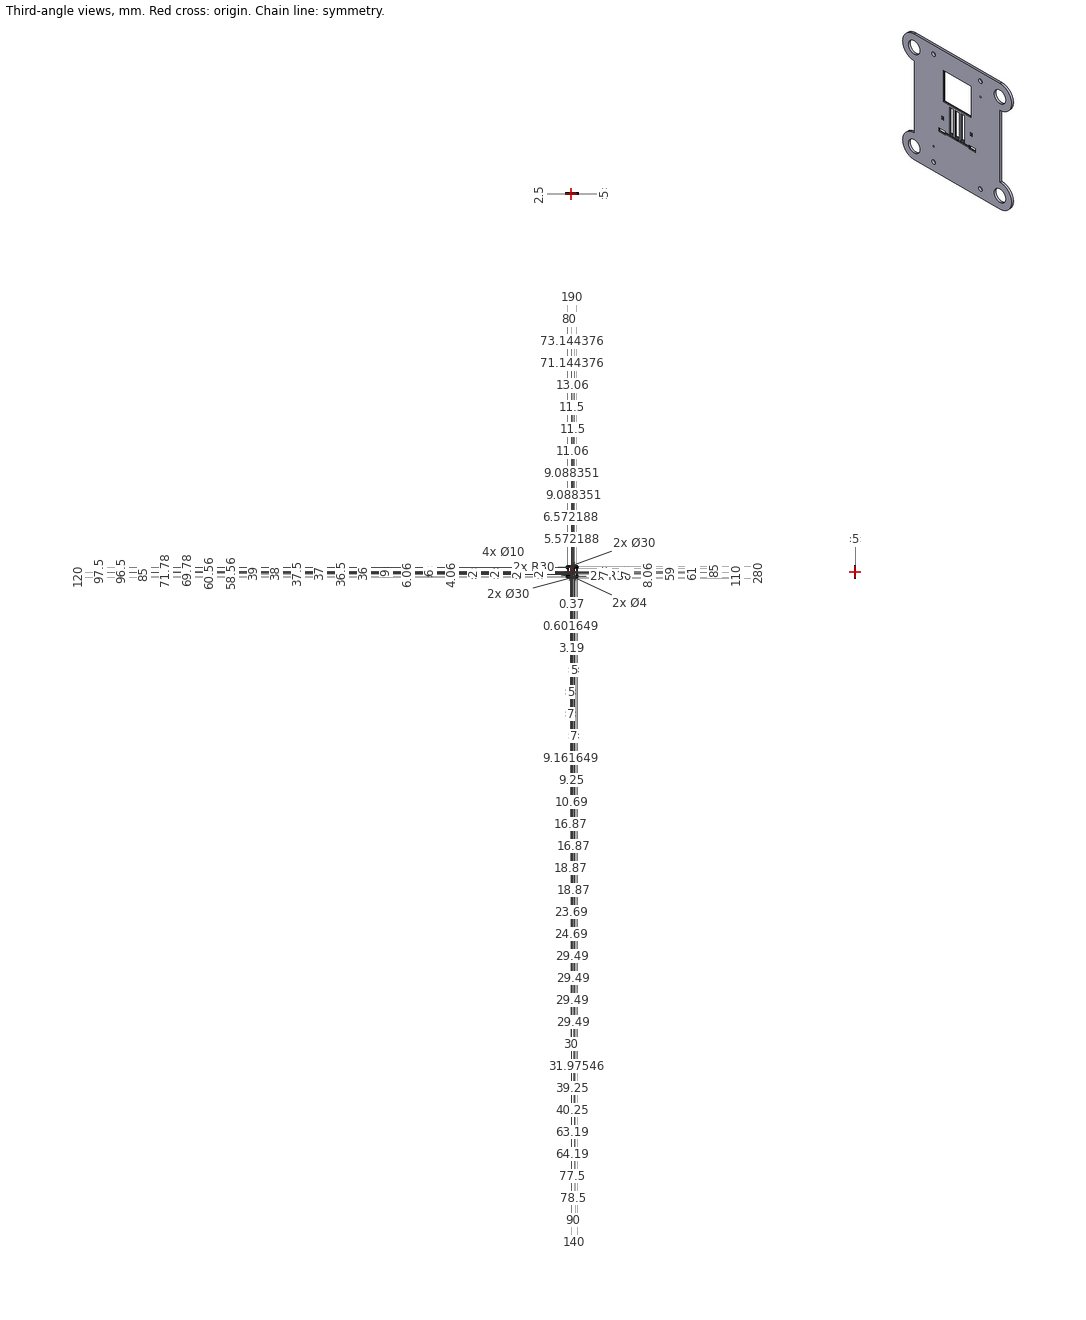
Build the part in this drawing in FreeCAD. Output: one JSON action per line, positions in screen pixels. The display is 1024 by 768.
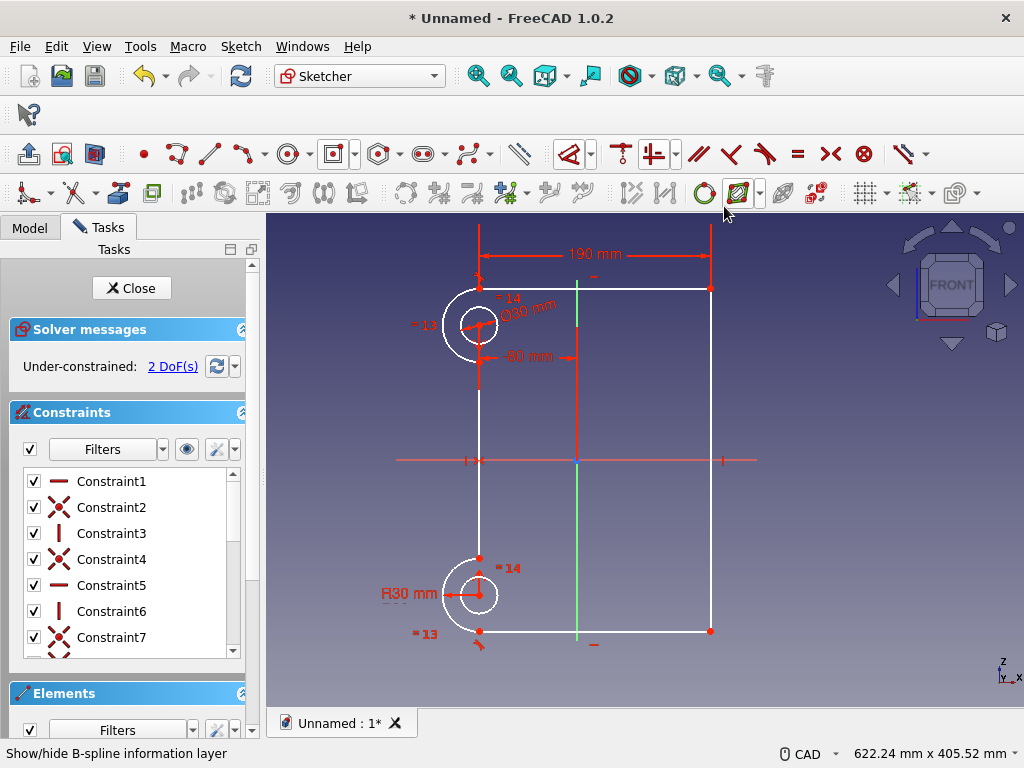
{"action": "left_click", "coordinate": [711, 392]}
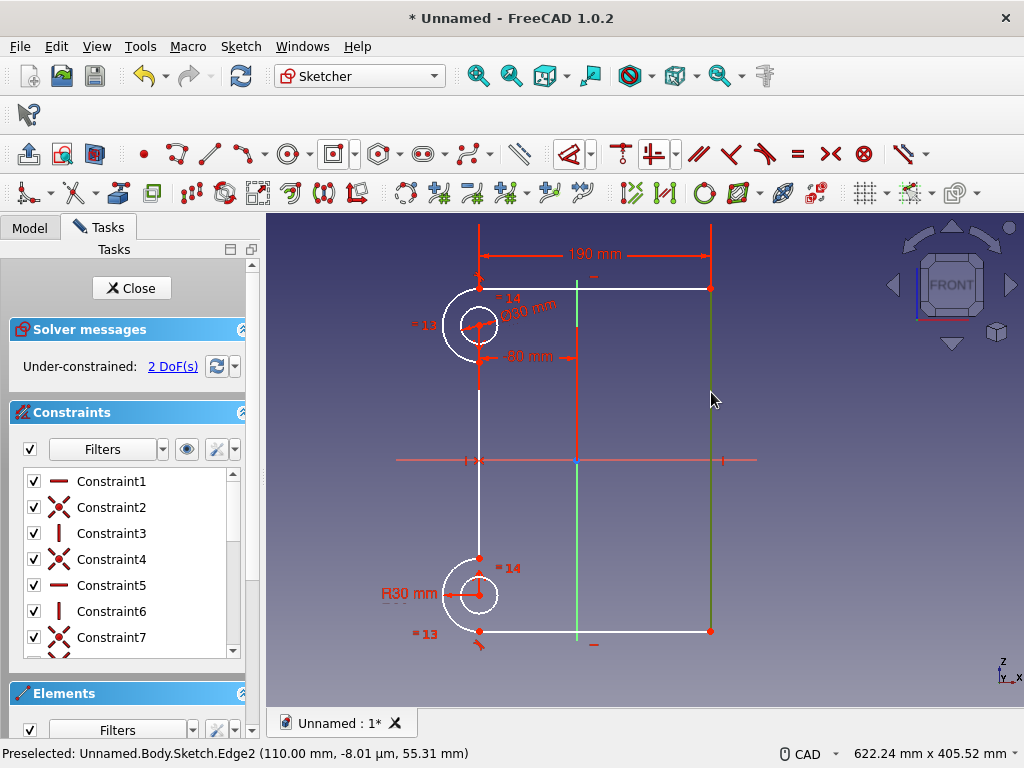
{"action": "left_click", "coordinate": [590, 154]}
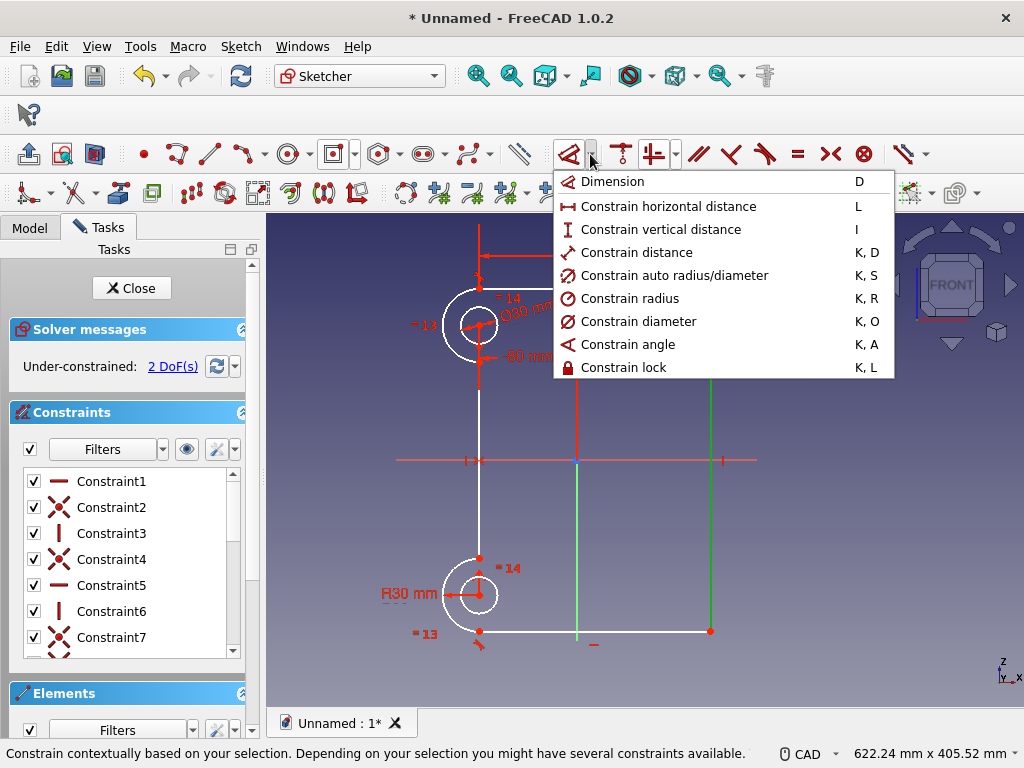
{"action": "left_click", "coordinate": [724, 230]}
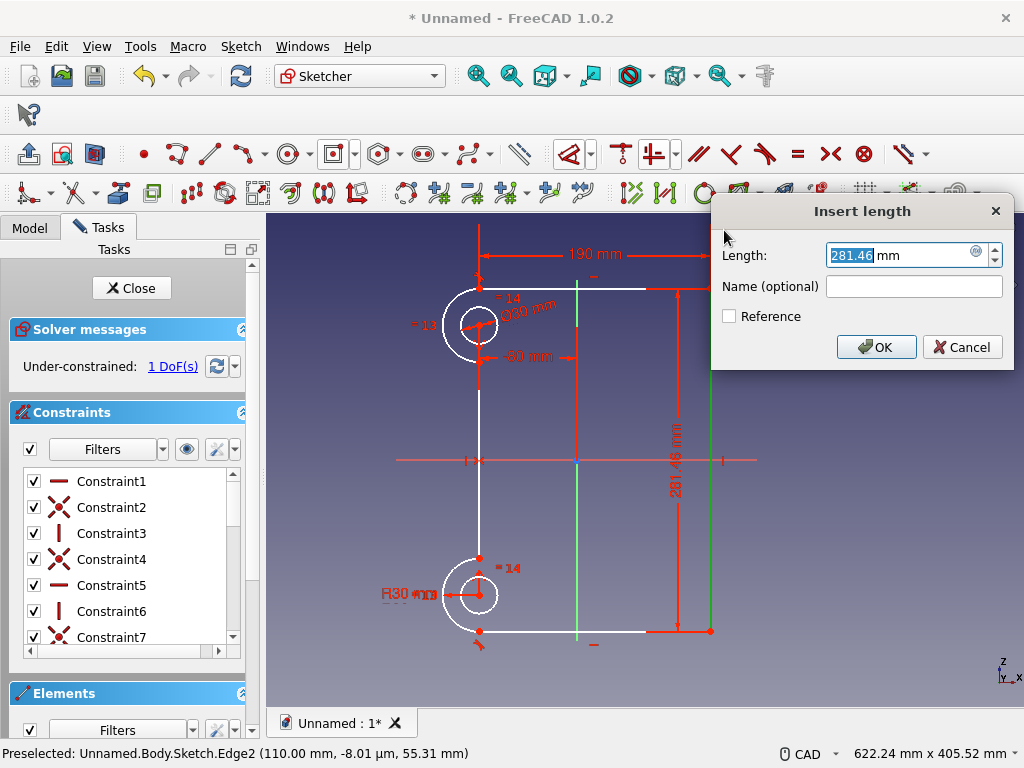
{"action": "type", "text": "280"}
{"action": "key", "text": "Return"}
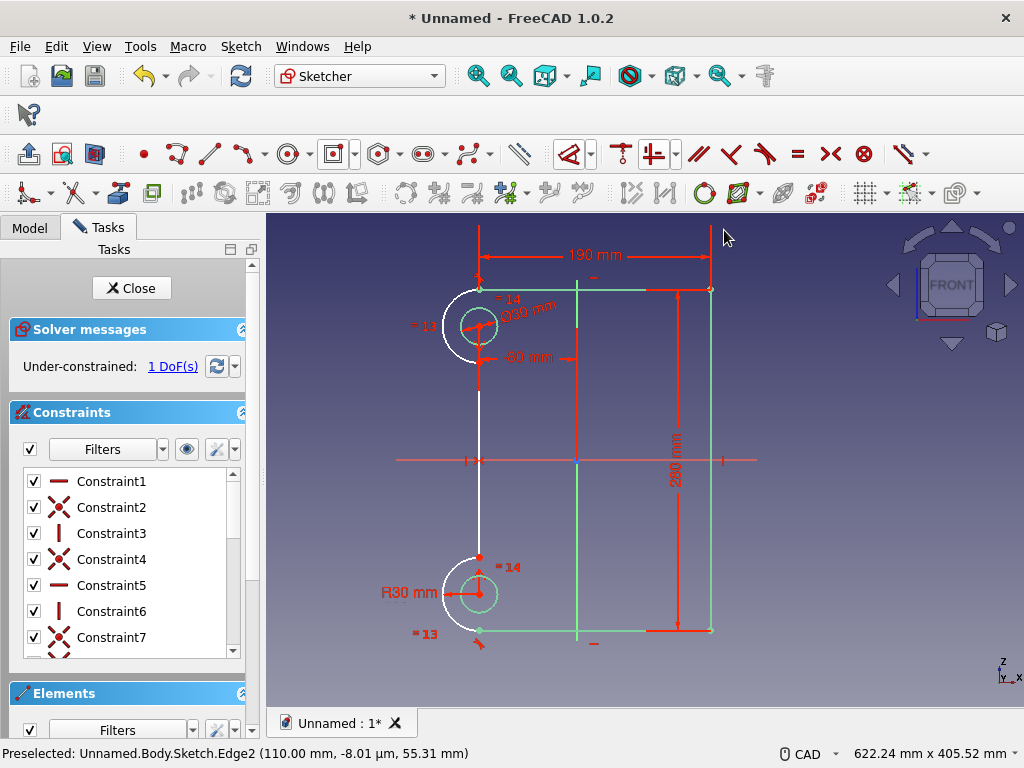
{"action": "left_click", "coordinate": [479, 558]}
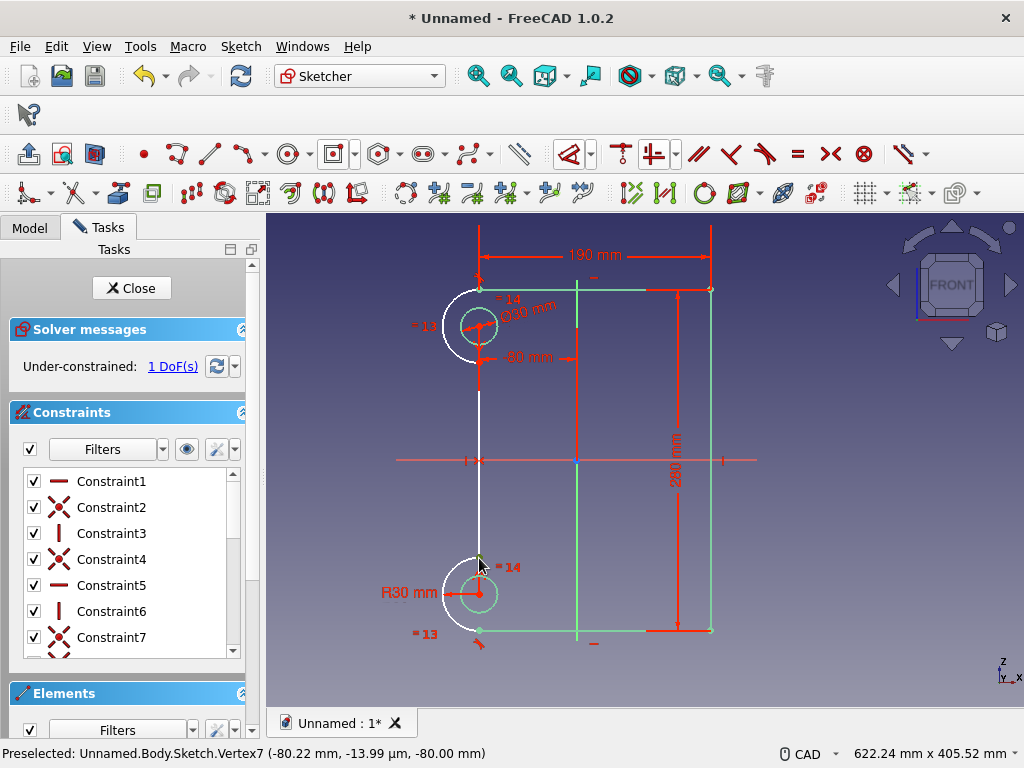
{"action": "left_click", "coordinate": [590, 154]}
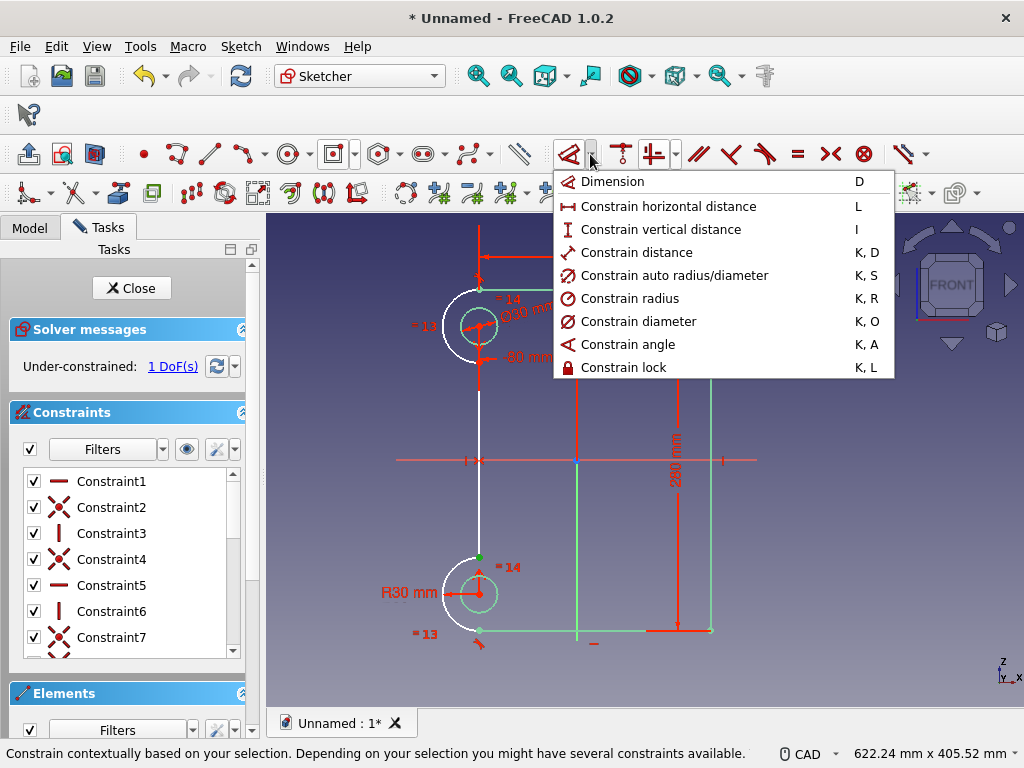
{"action": "left_click", "coordinate": [724, 206]}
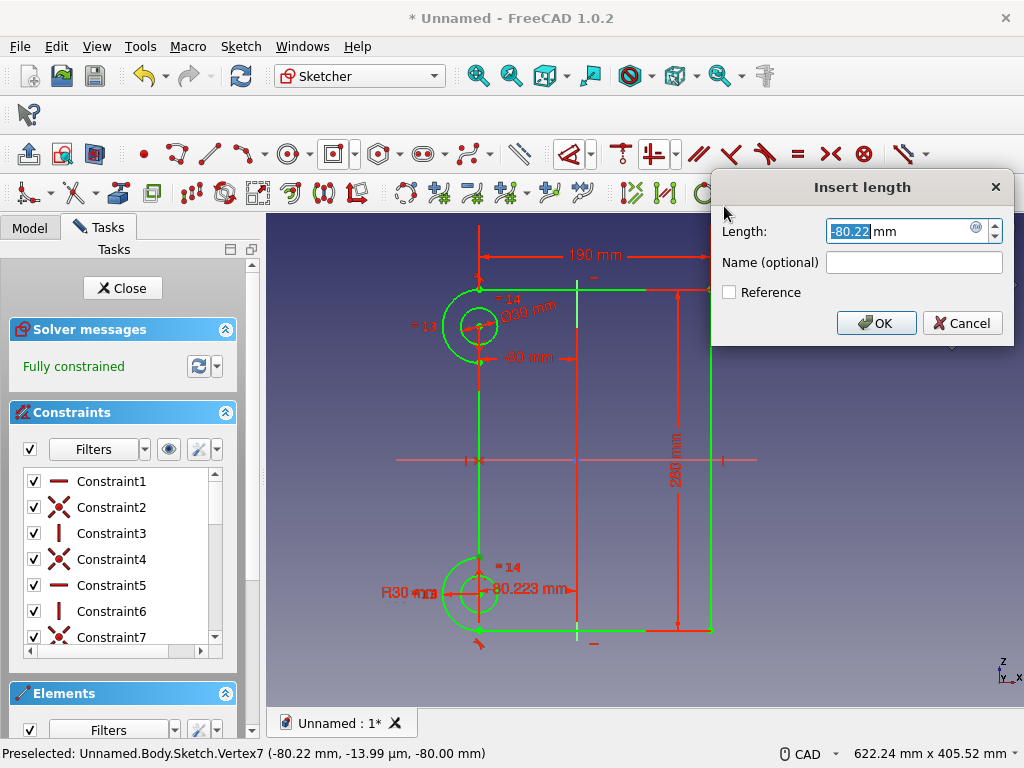
{"action": "type", "text": "-80"}
{"action": "key", "text": "Return"}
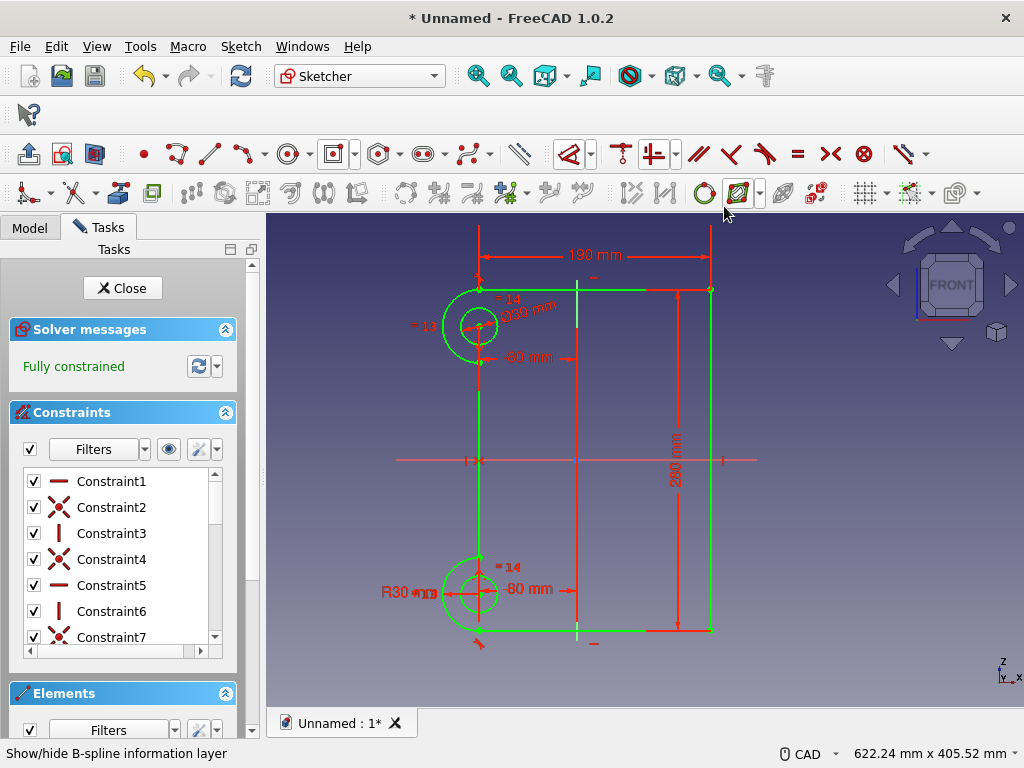
{"action": "left_click", "coordinate": [123, 288]}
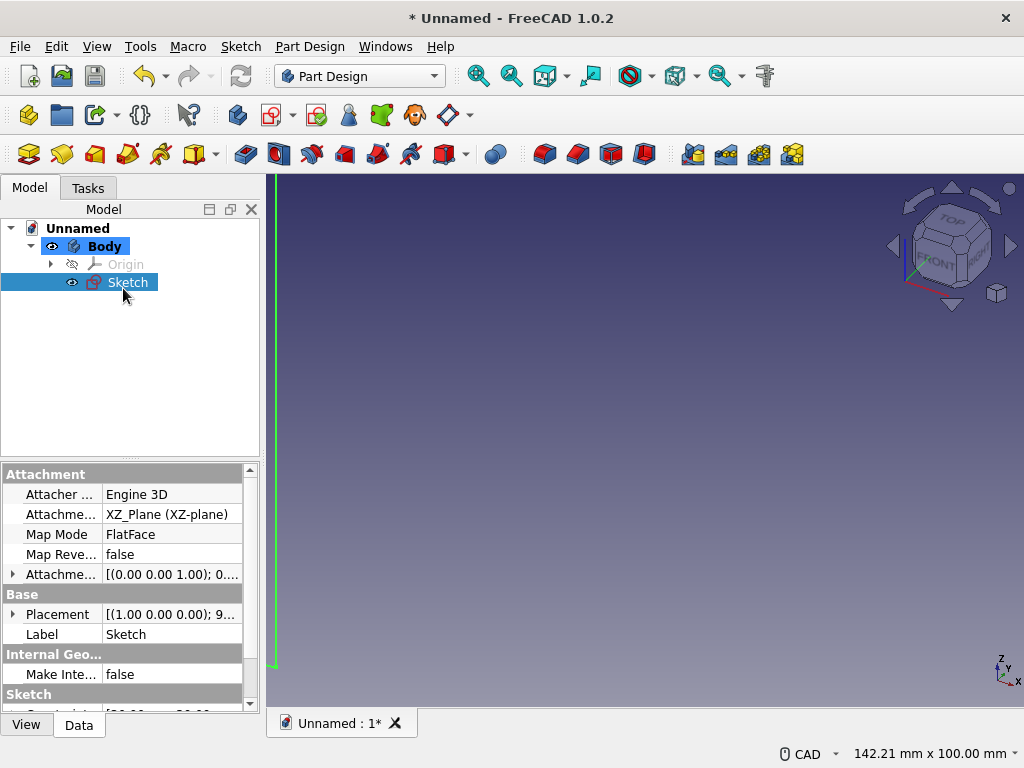
{"action": "left_click", "coordinate": [29, 154]}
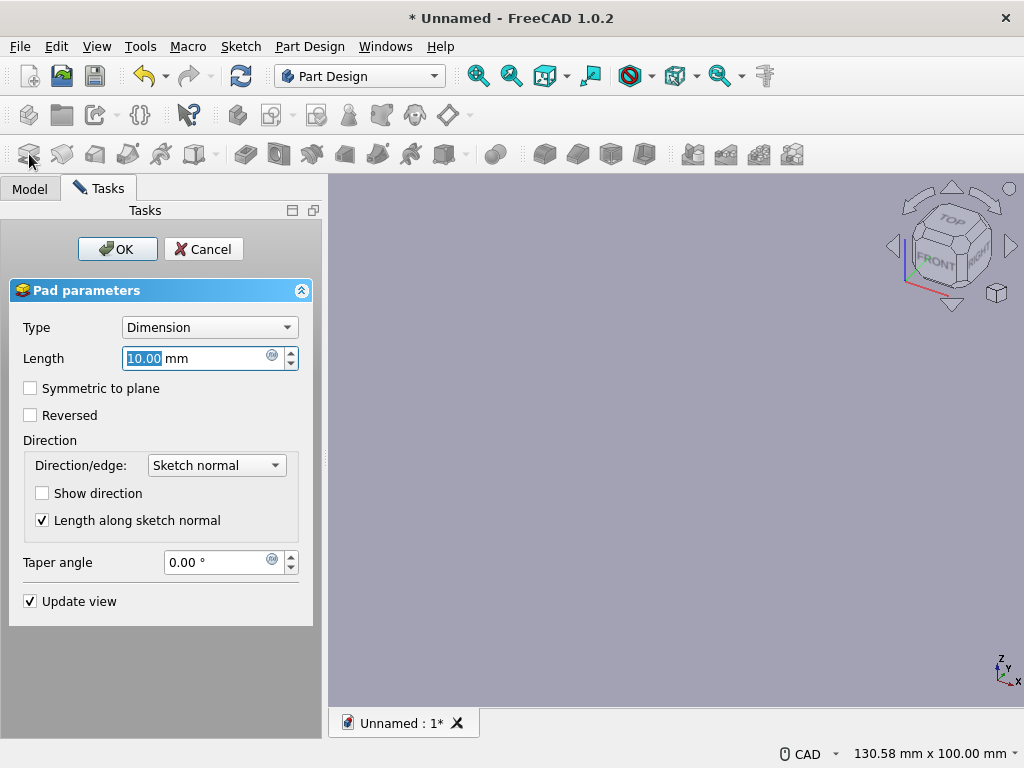
{"action": "type", "text": "5"}
{"action": "key", "text": "Tab"}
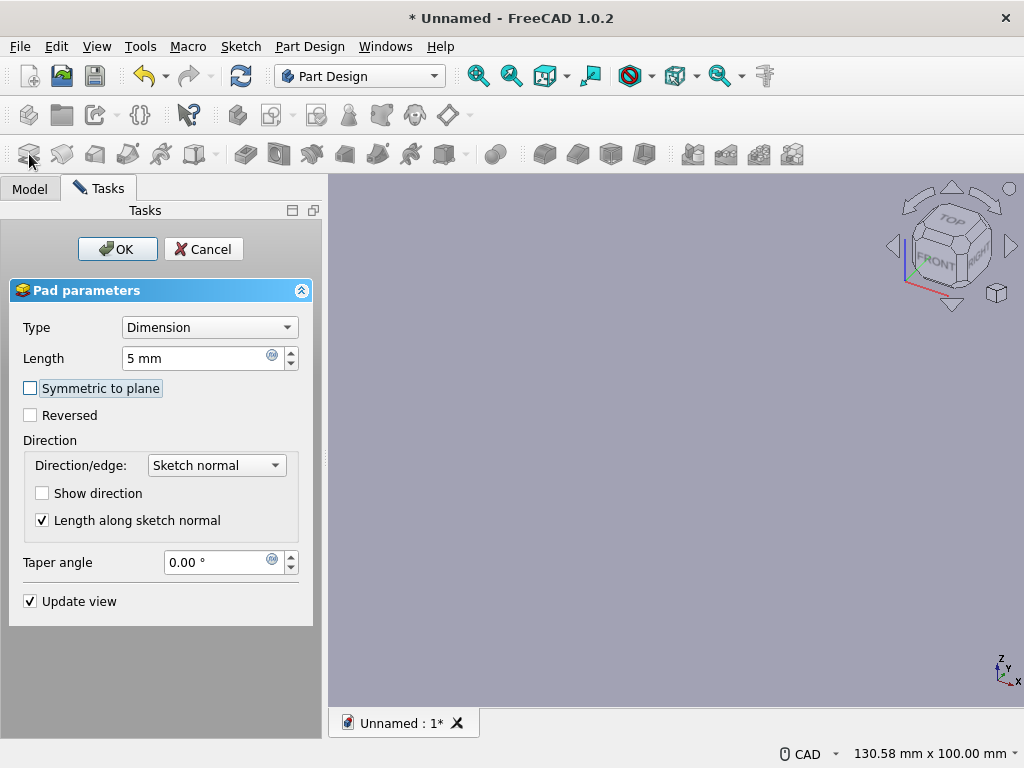
{"action": "left_click", "coordinate": [31, 415]}